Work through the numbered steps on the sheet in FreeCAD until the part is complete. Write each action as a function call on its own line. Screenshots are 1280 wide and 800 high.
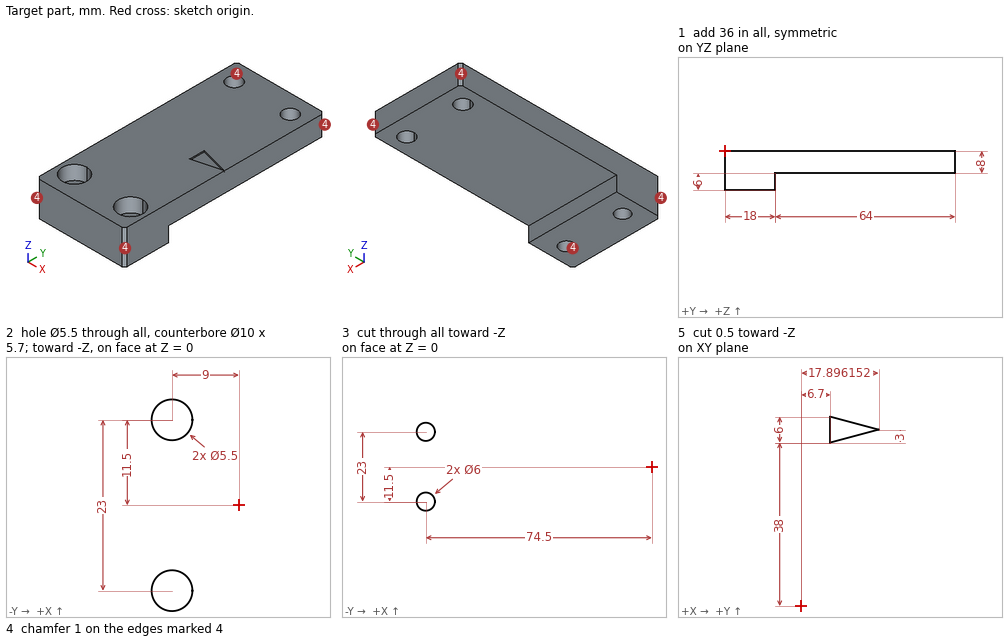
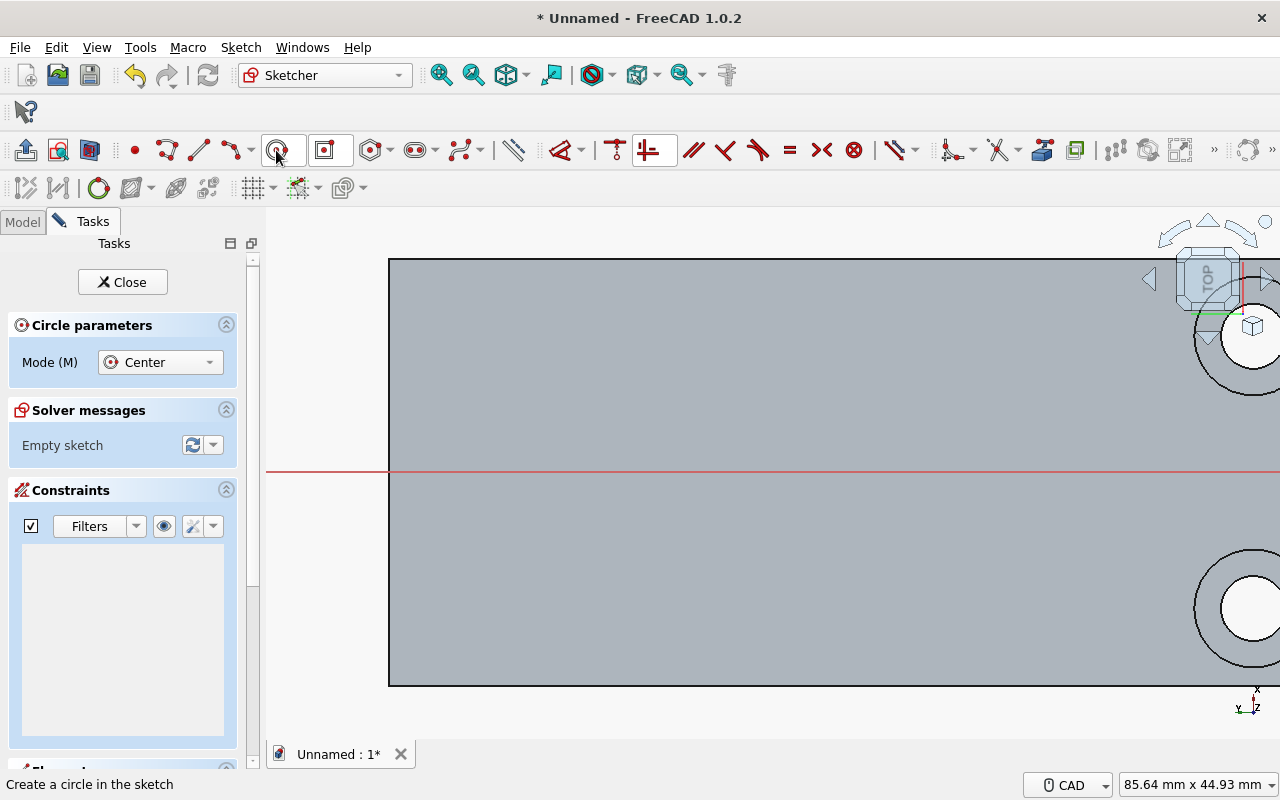
click(478, 609)
move(503, 583)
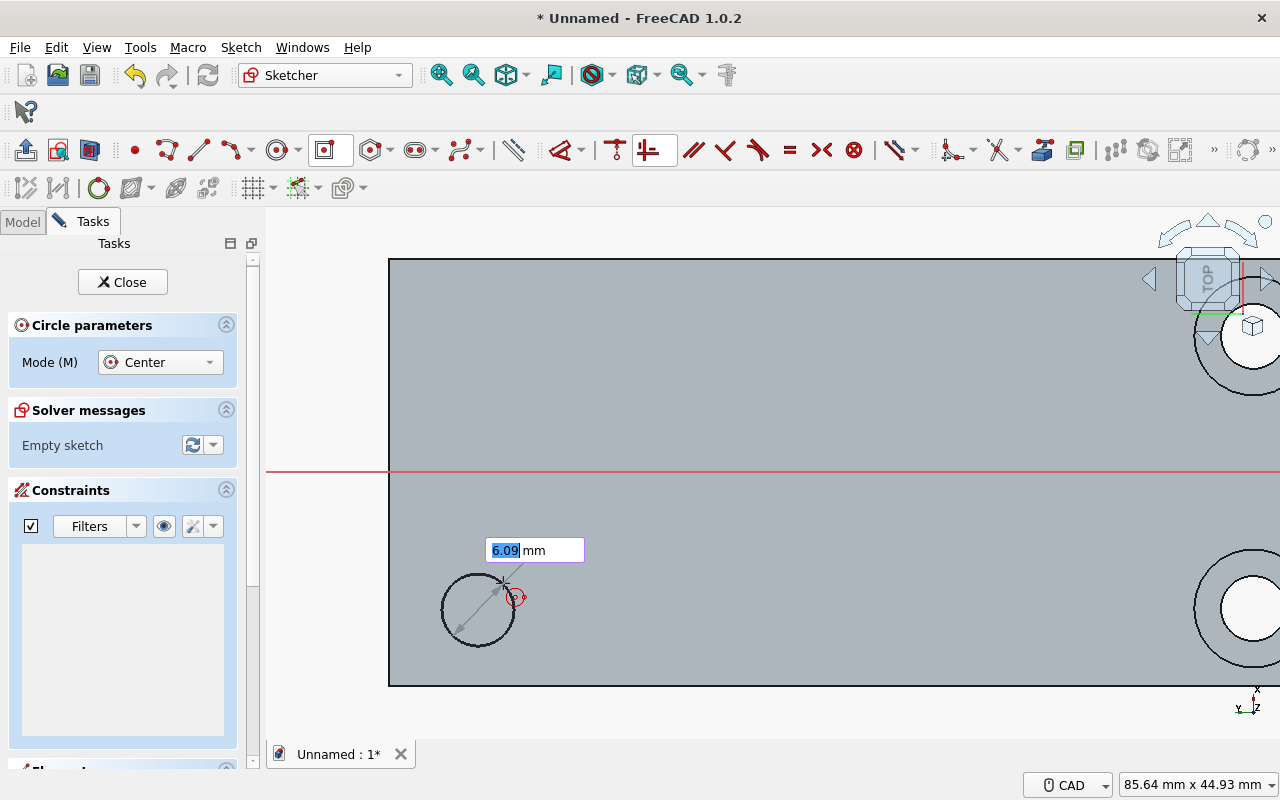
text(6)
key(Return)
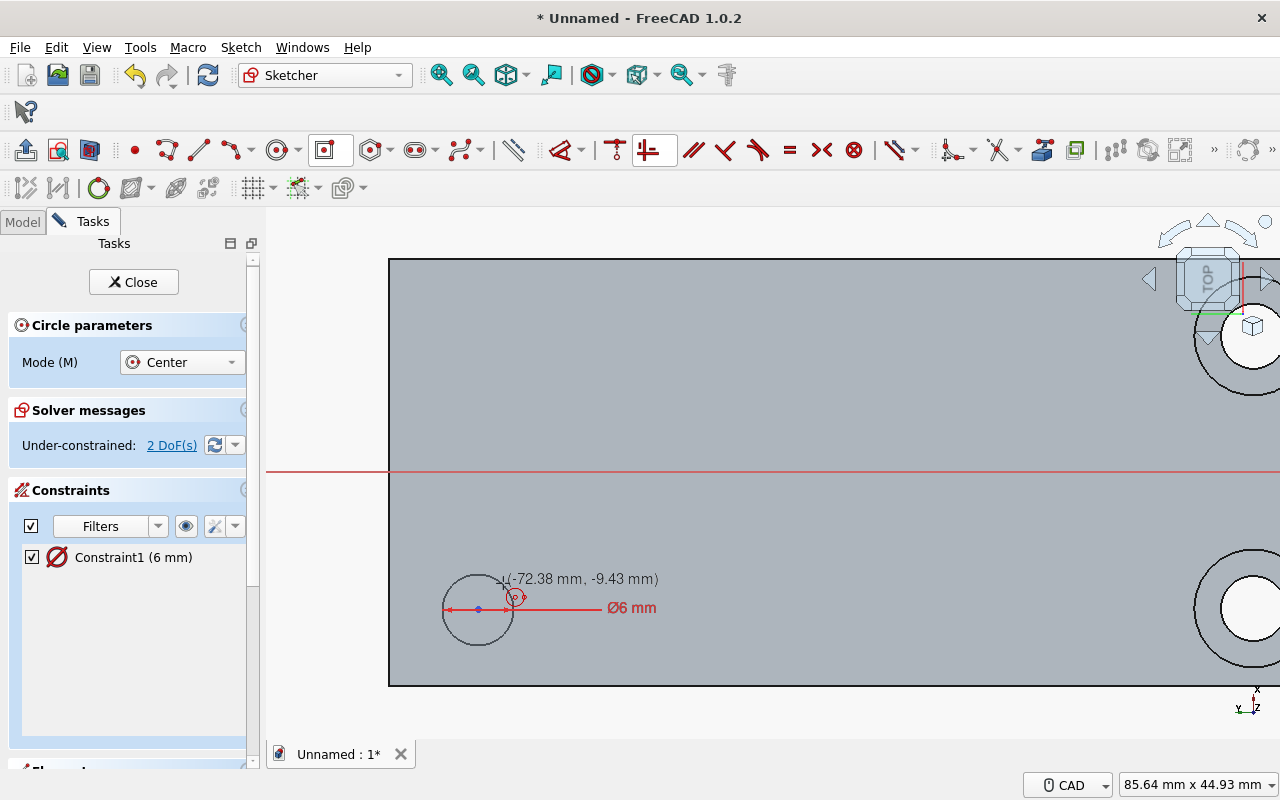
click(478, 336)
move(503, 311)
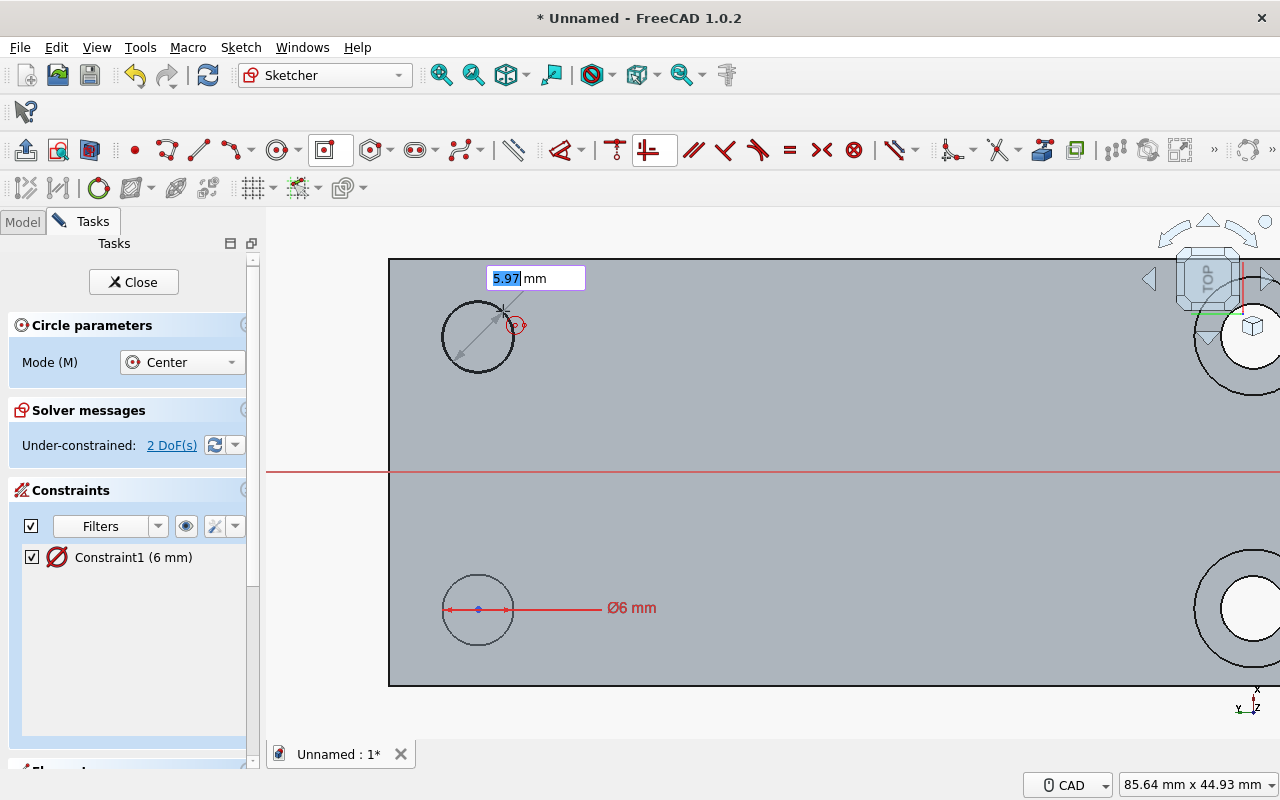
text(6)
key(Return)
key(Escape)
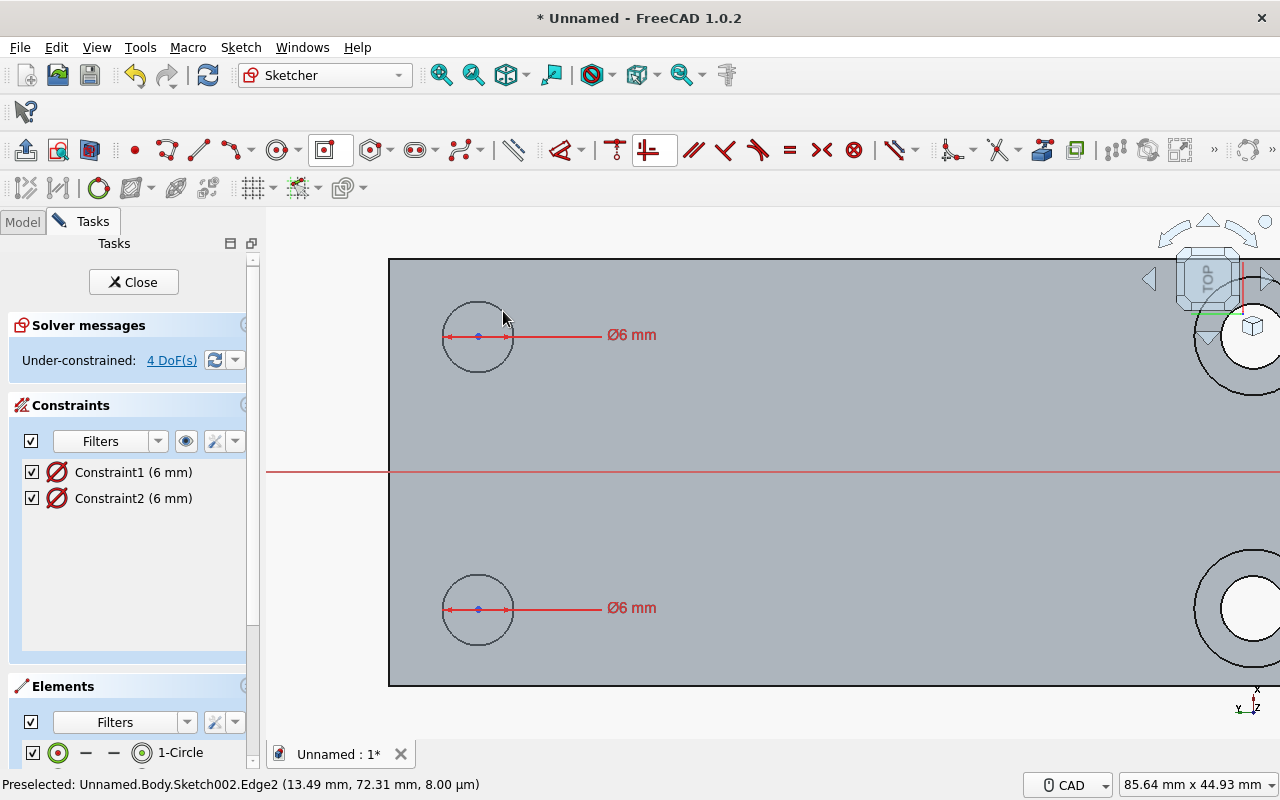
click(478, 610)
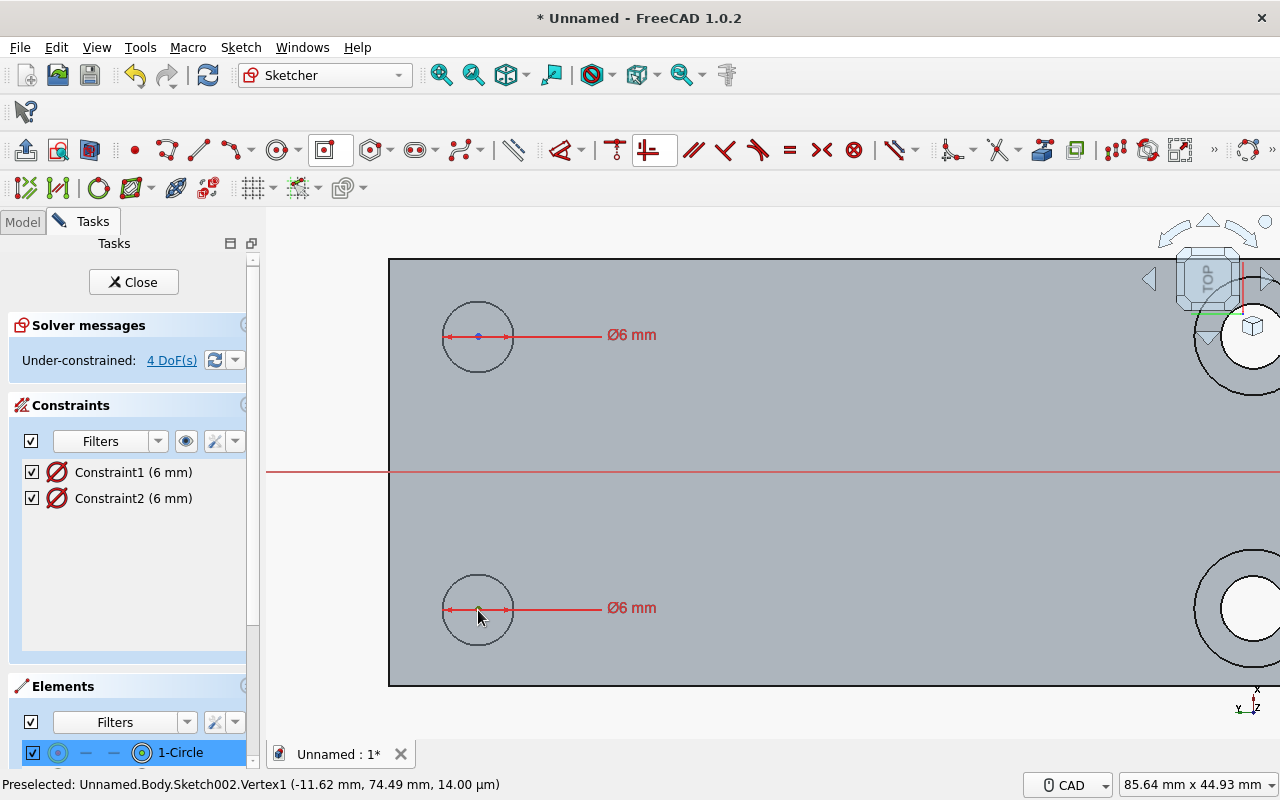
click(478, 337)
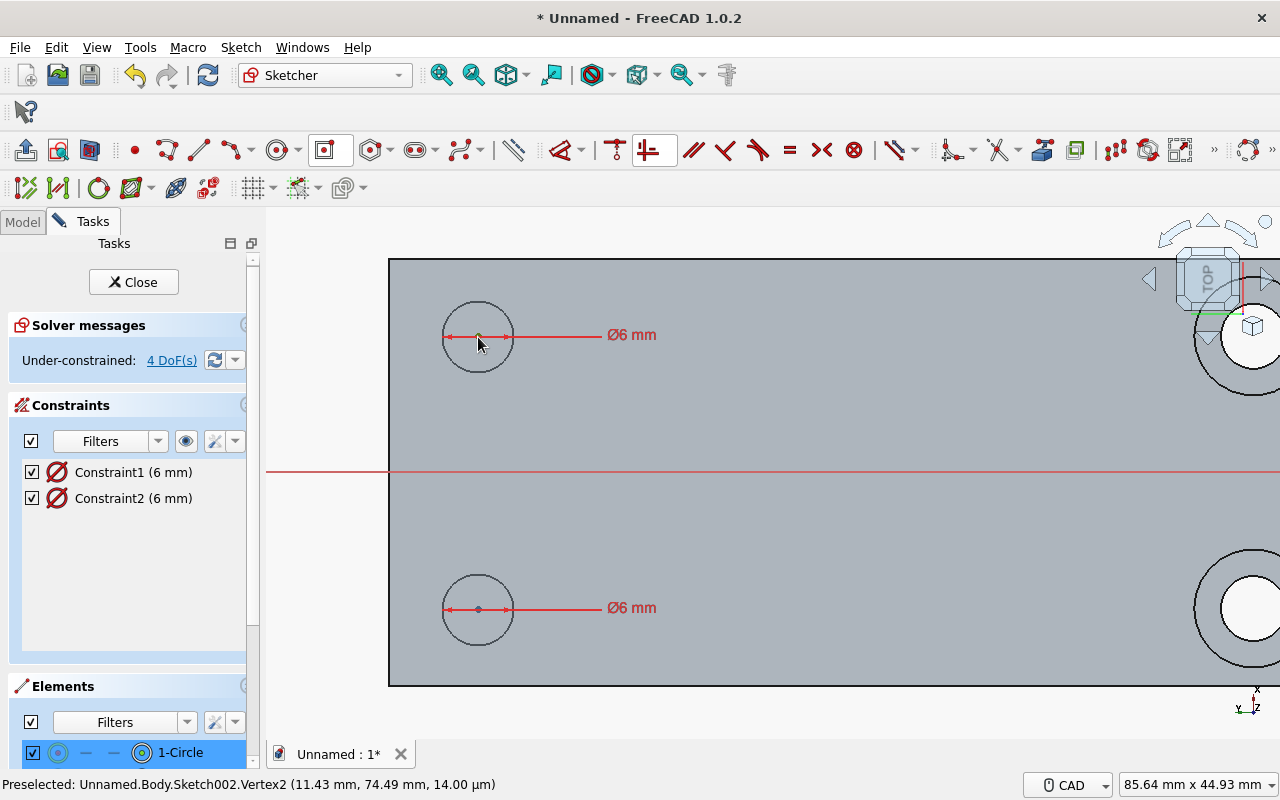
click(672, 150)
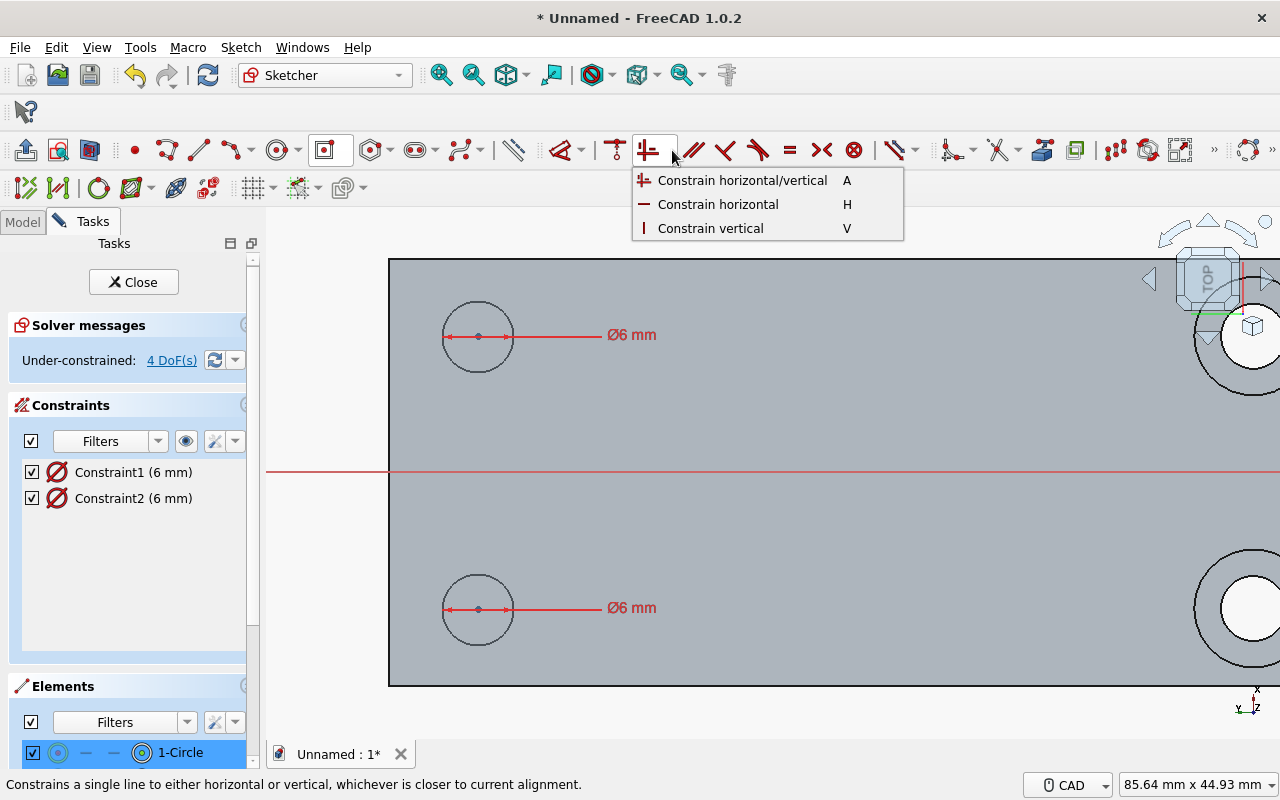
click(768, 228)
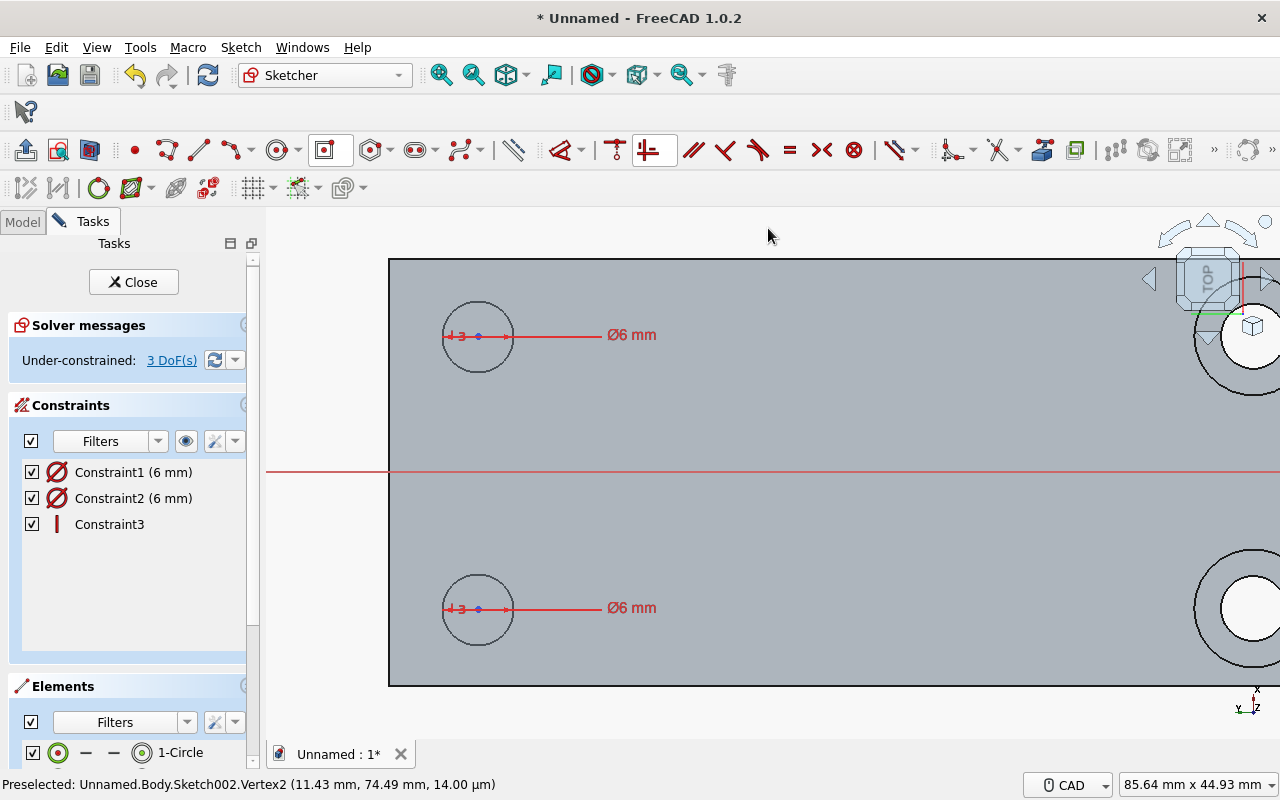
click(560, 150)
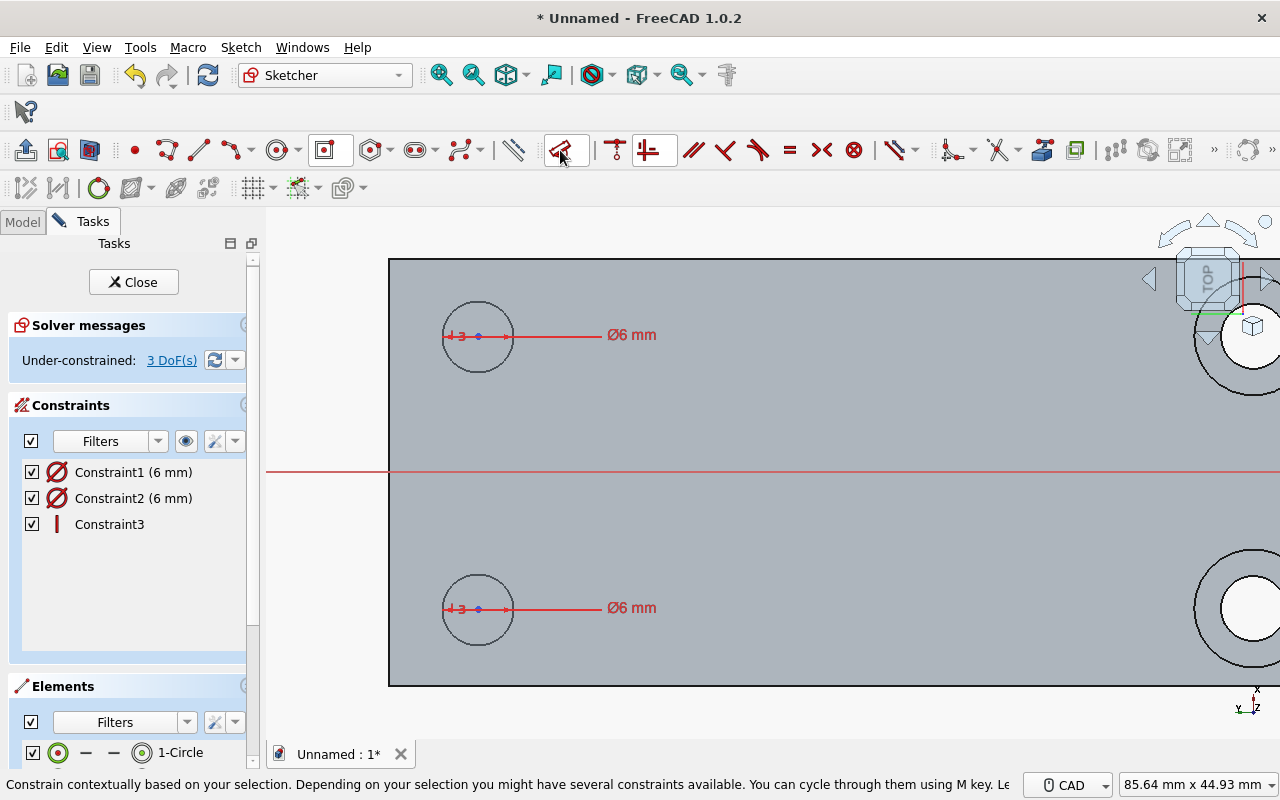
click(478, 610)